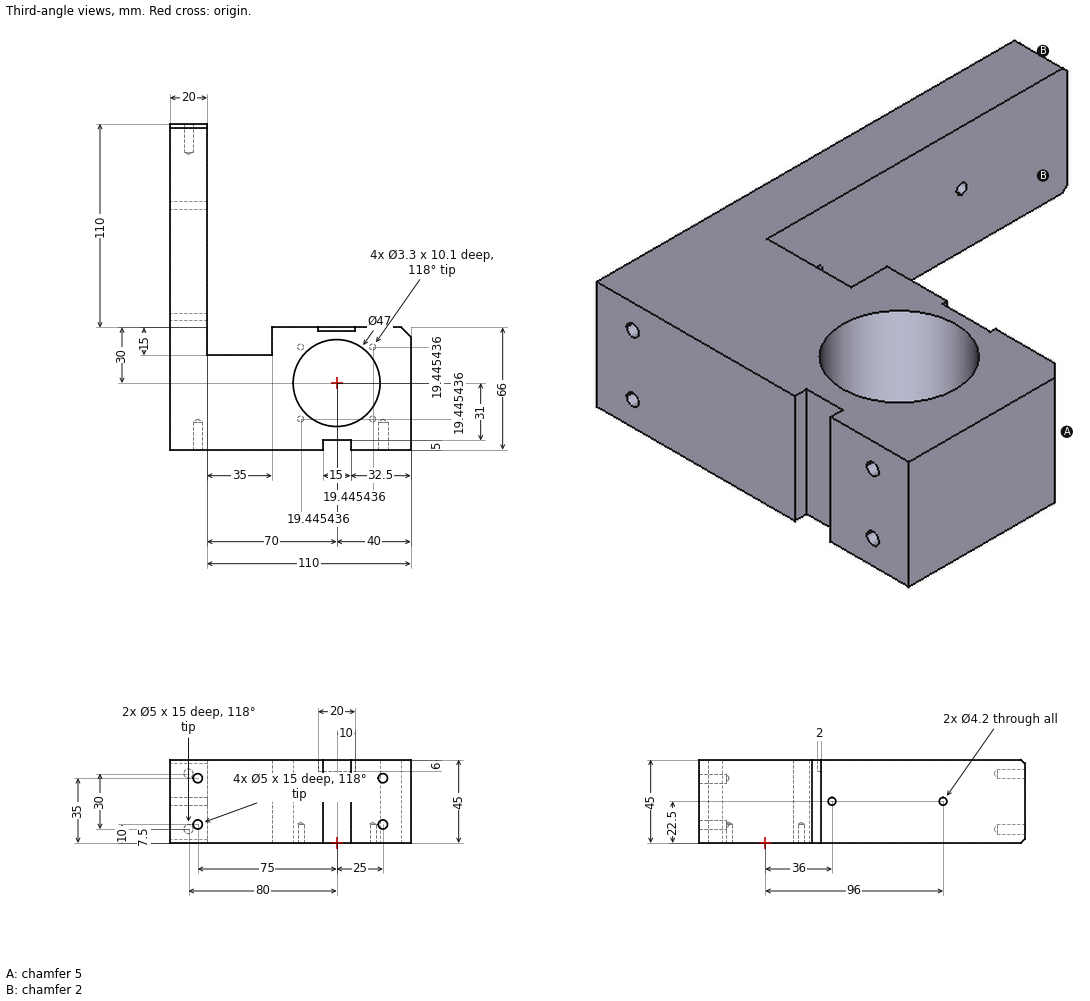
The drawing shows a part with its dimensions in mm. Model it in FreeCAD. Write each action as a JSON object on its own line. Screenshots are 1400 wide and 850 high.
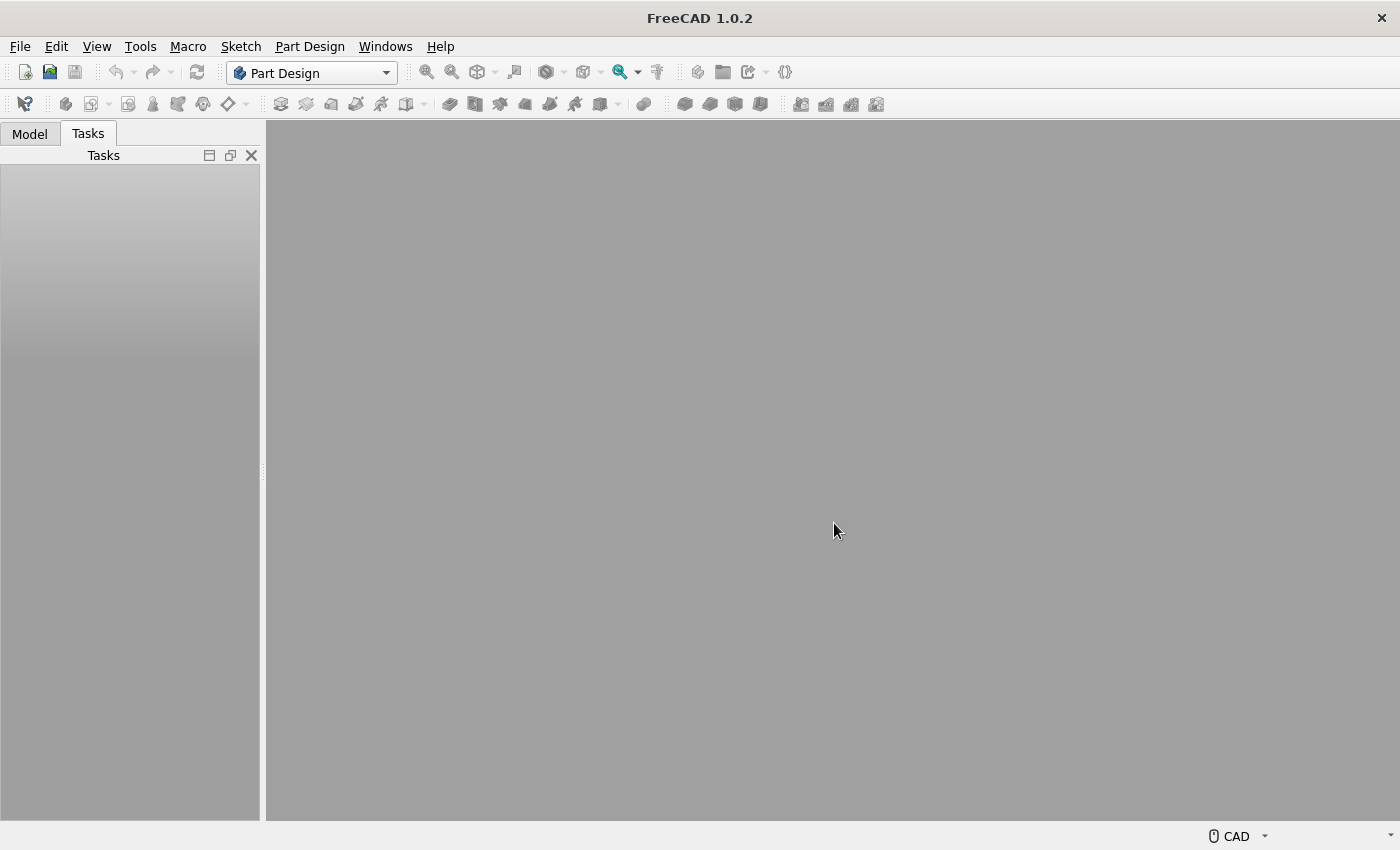
{"action": "left_click", "coordinate": [25, 72]}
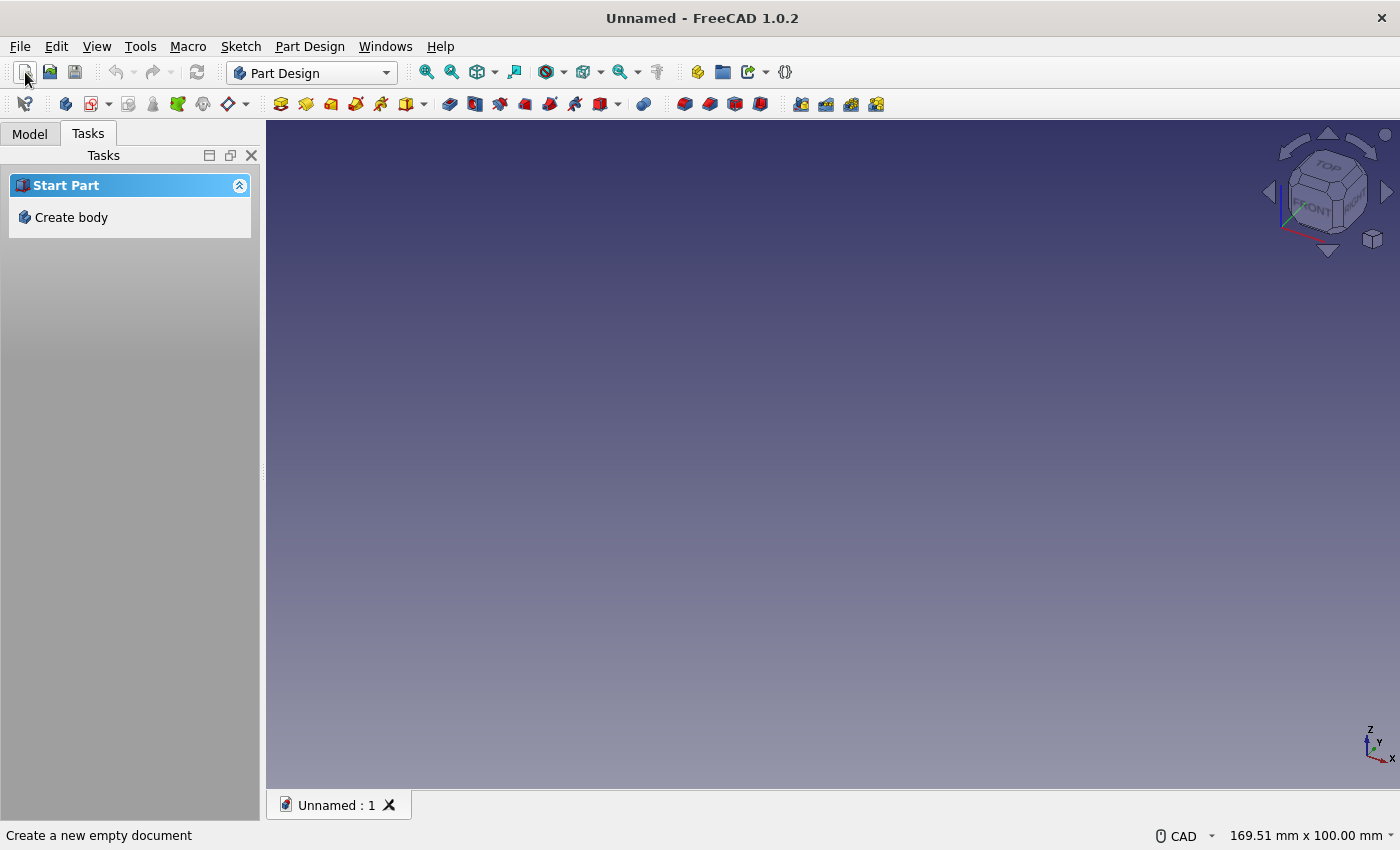
{"action": "left_click", "coordinate": [90, 104]}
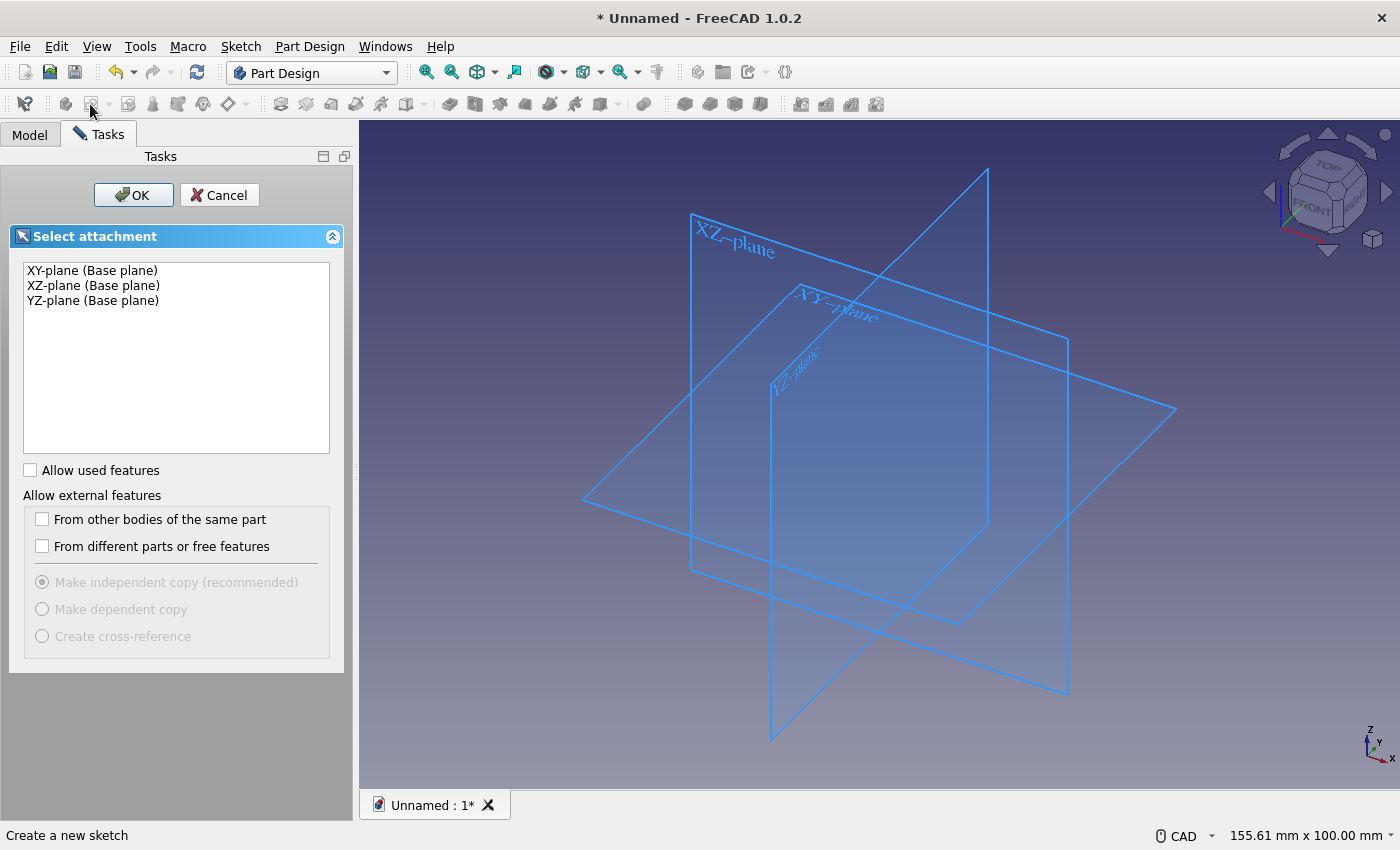
{"action": "left_click", "coordinate": [84, 270]}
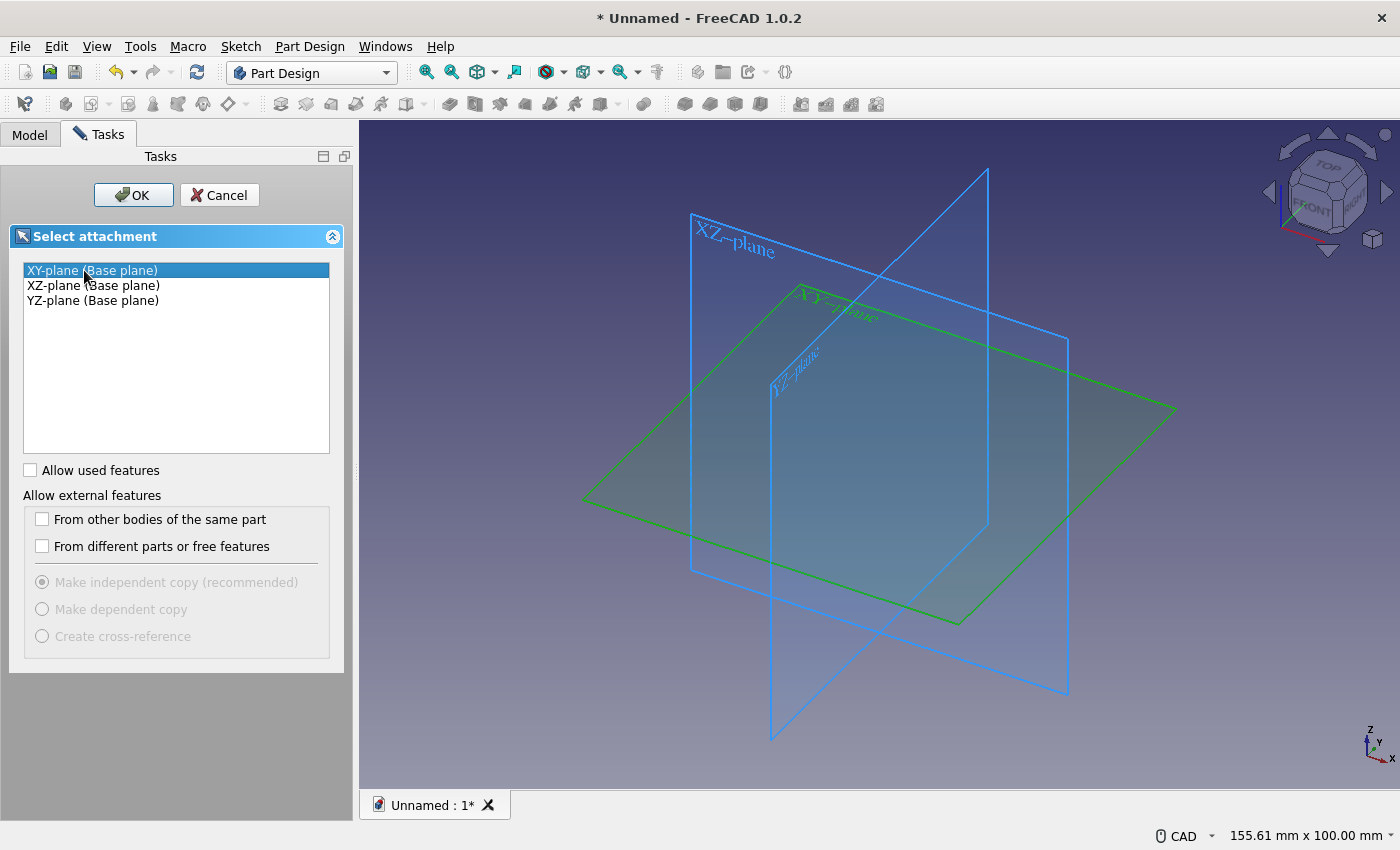
{"action": "left_click", "coordinate": [134, 195]}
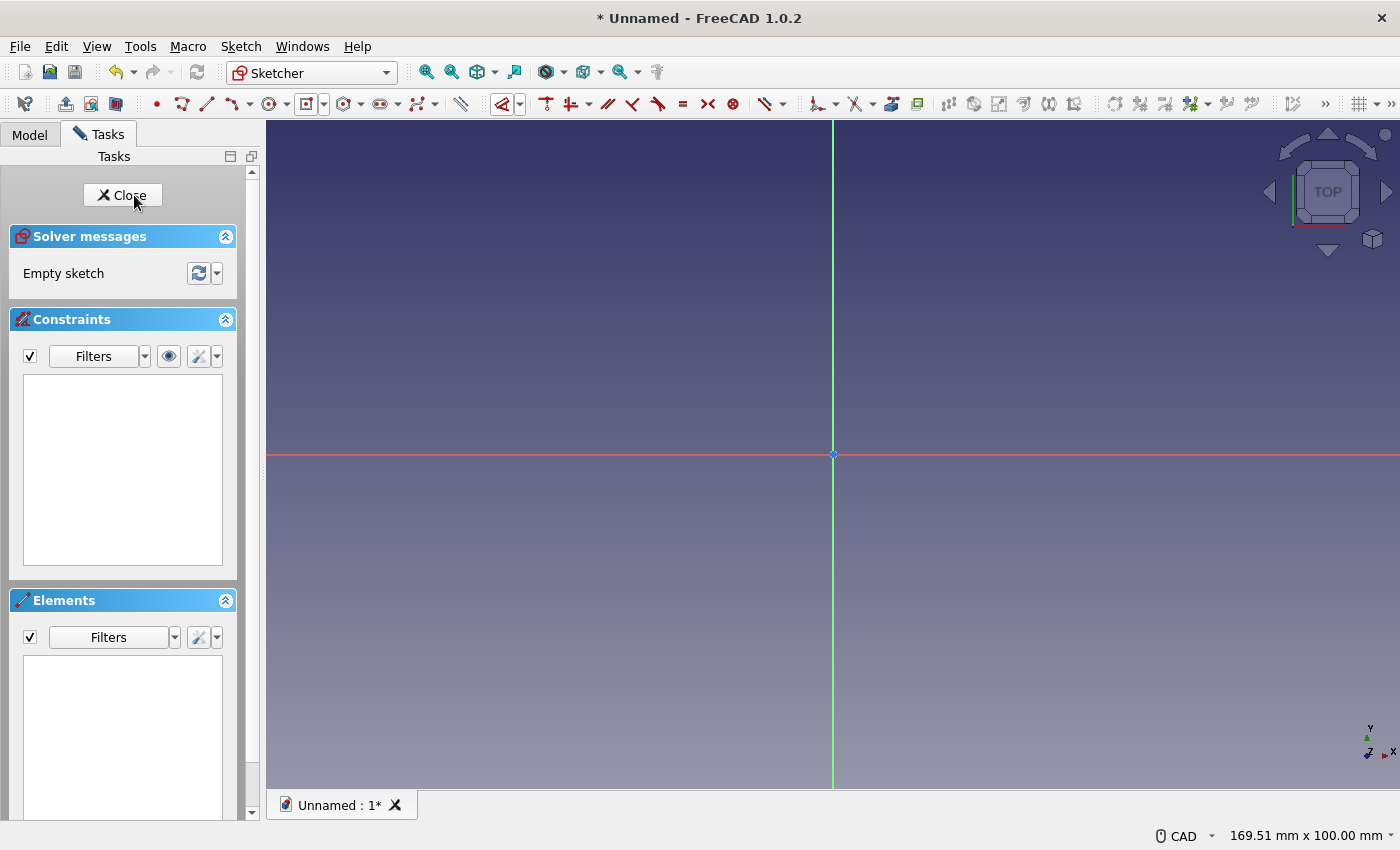
{"action": "scroll", "coordinate": [822, 657], "scroll_direction": "down", "scroll_amount": 5}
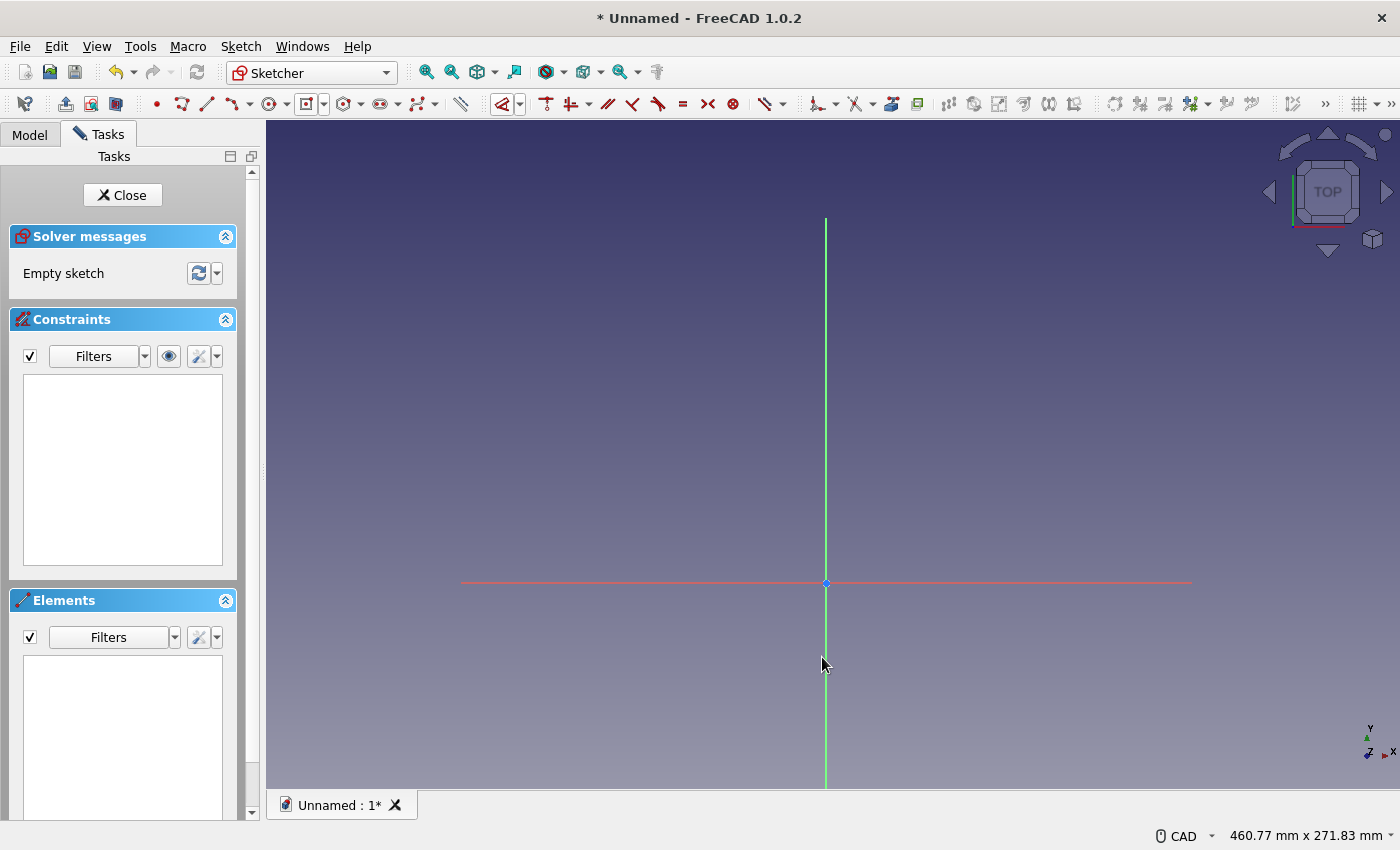
{"action": "key", "text": "g m"}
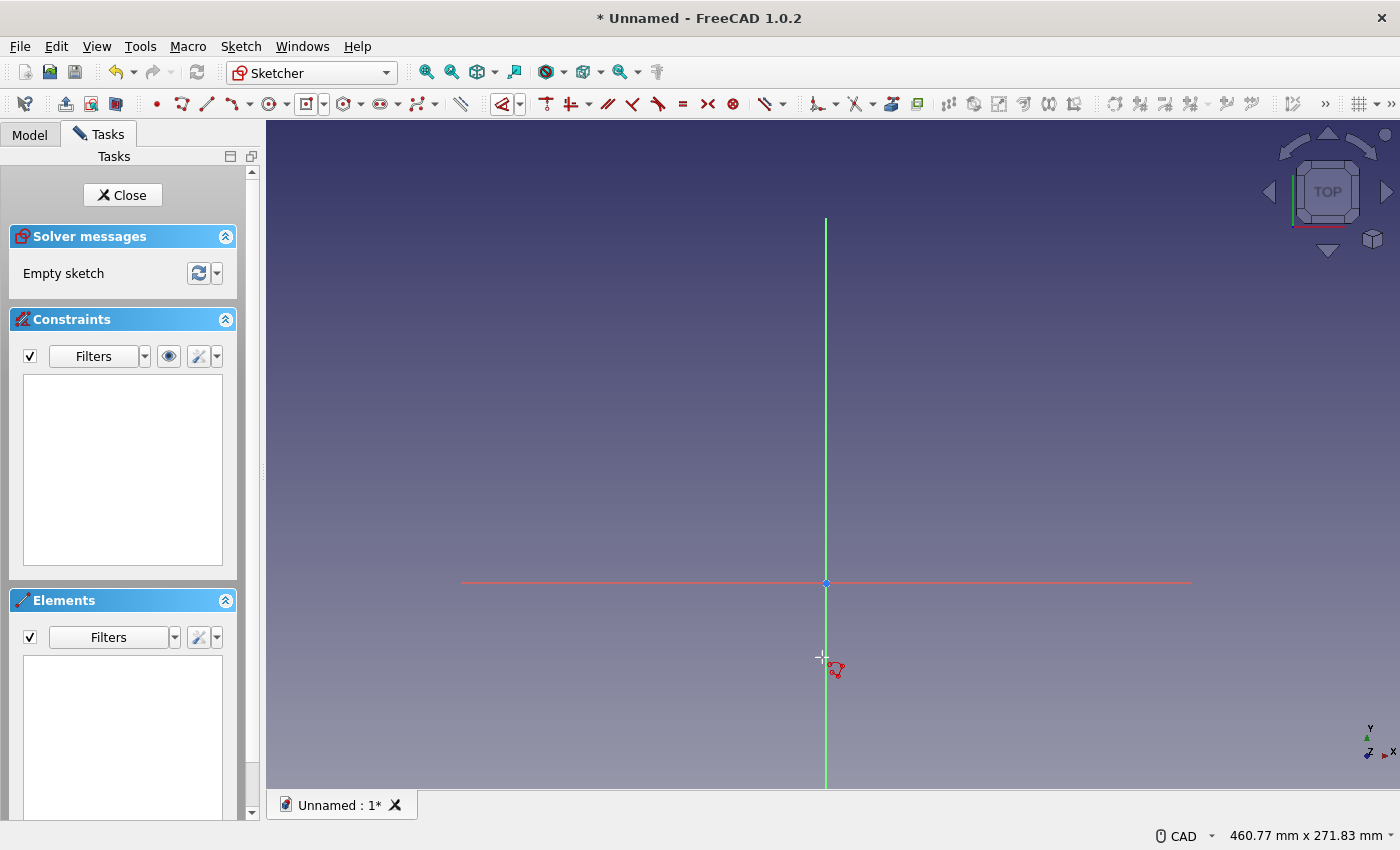
{"action": "left_click", "coordinate": [808, 659]}
{"action": "left_click", "coordinate": [845, 659]}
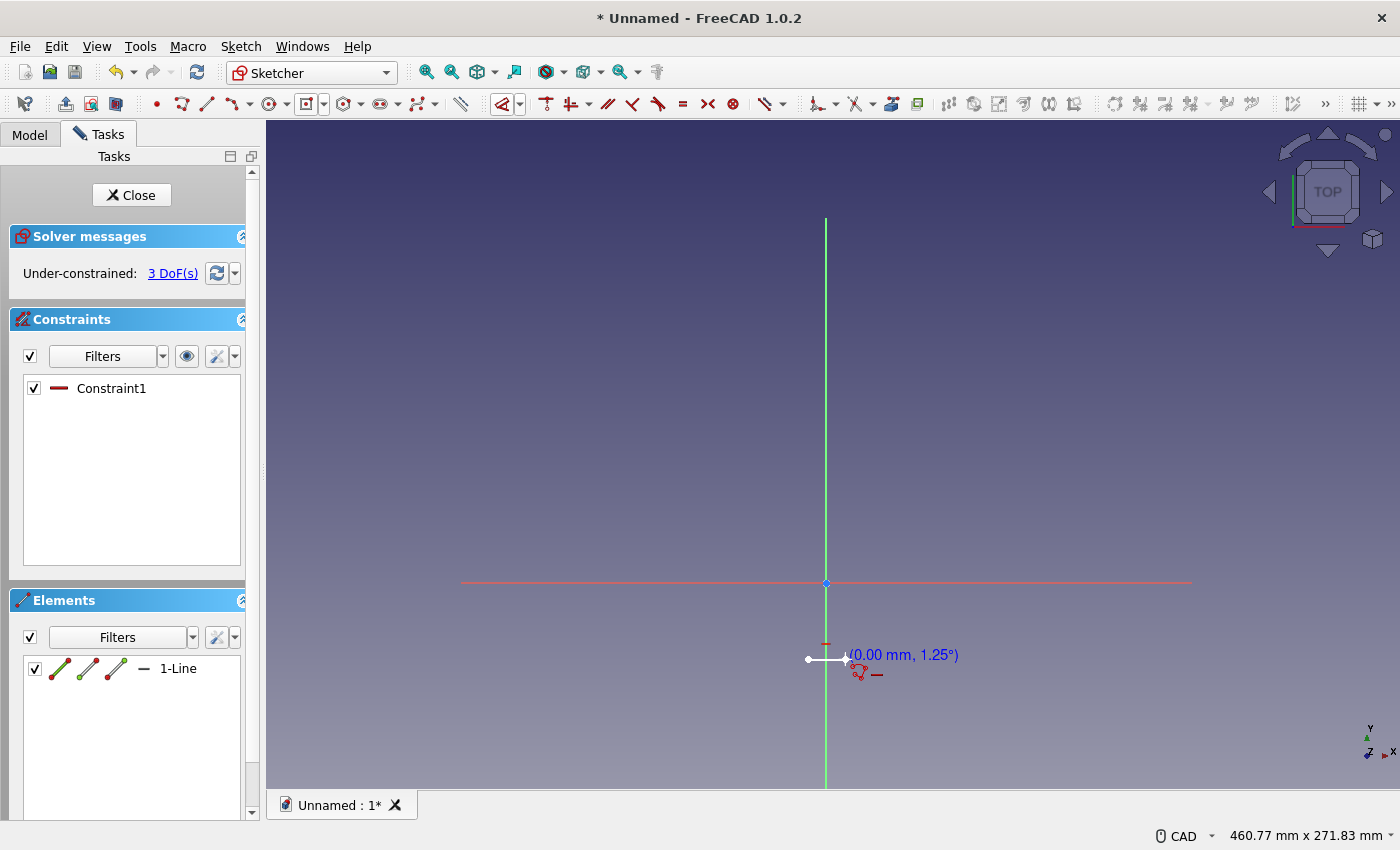
{"action": "scroll", "coordinate": [845, 672], "scroll_direction": "up", "scroll_amount": 2}